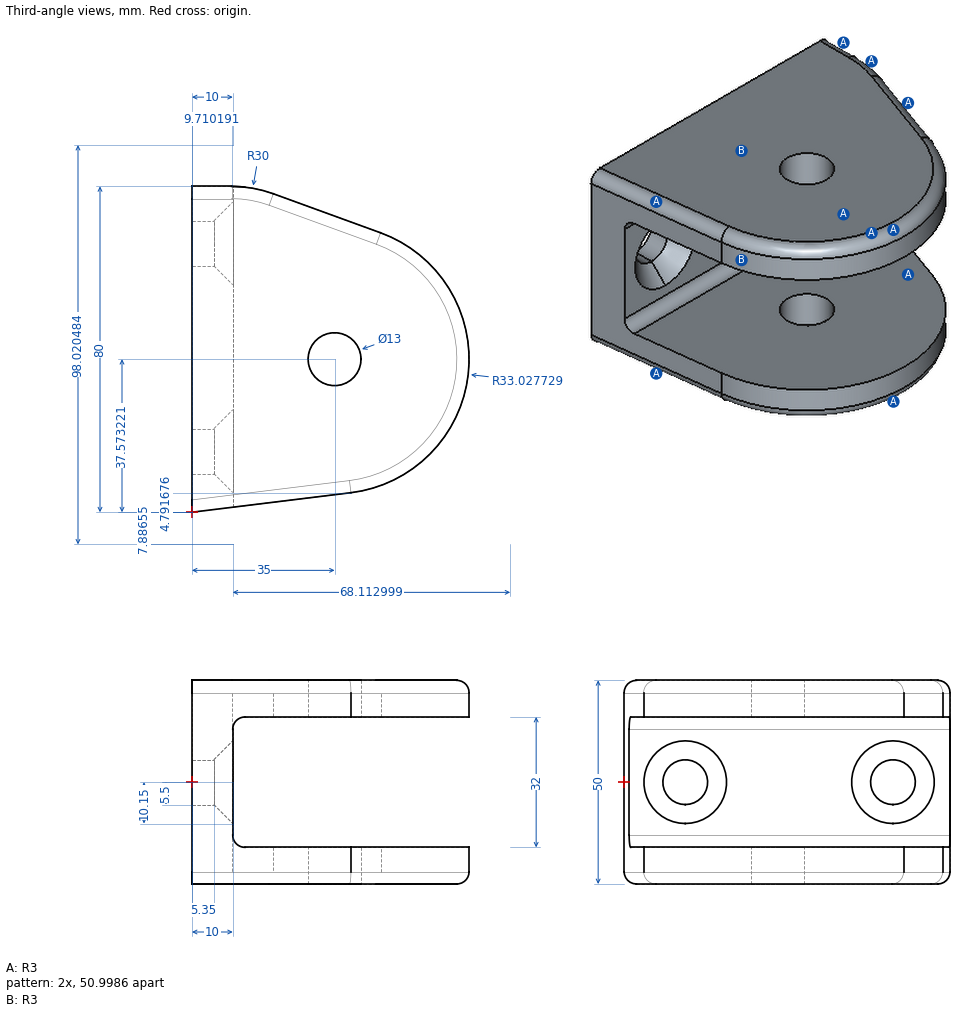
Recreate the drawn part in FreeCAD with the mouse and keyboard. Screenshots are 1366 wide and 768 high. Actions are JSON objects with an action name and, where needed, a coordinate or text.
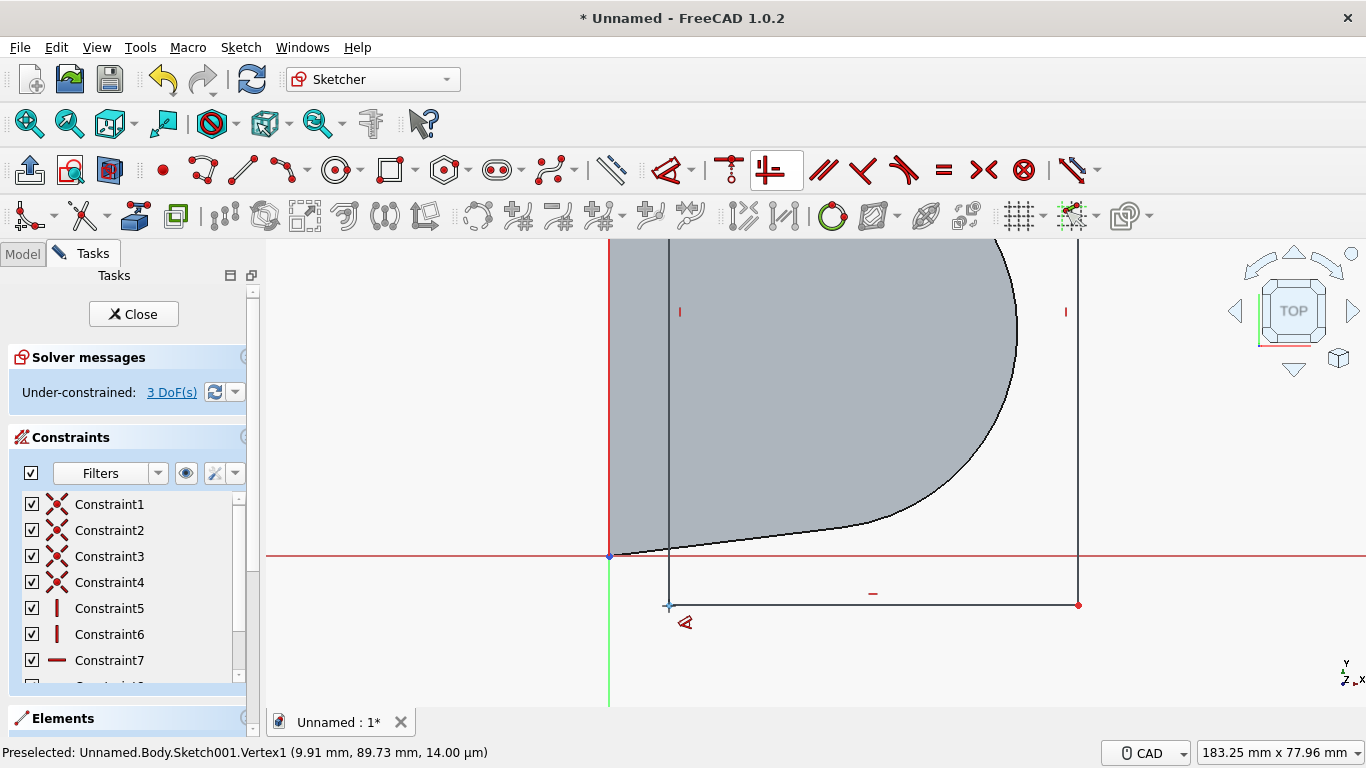
{"action": "left_click", "coordinate": [669, 605]}
{"action": "left_click", "coordinate": [575, 581]}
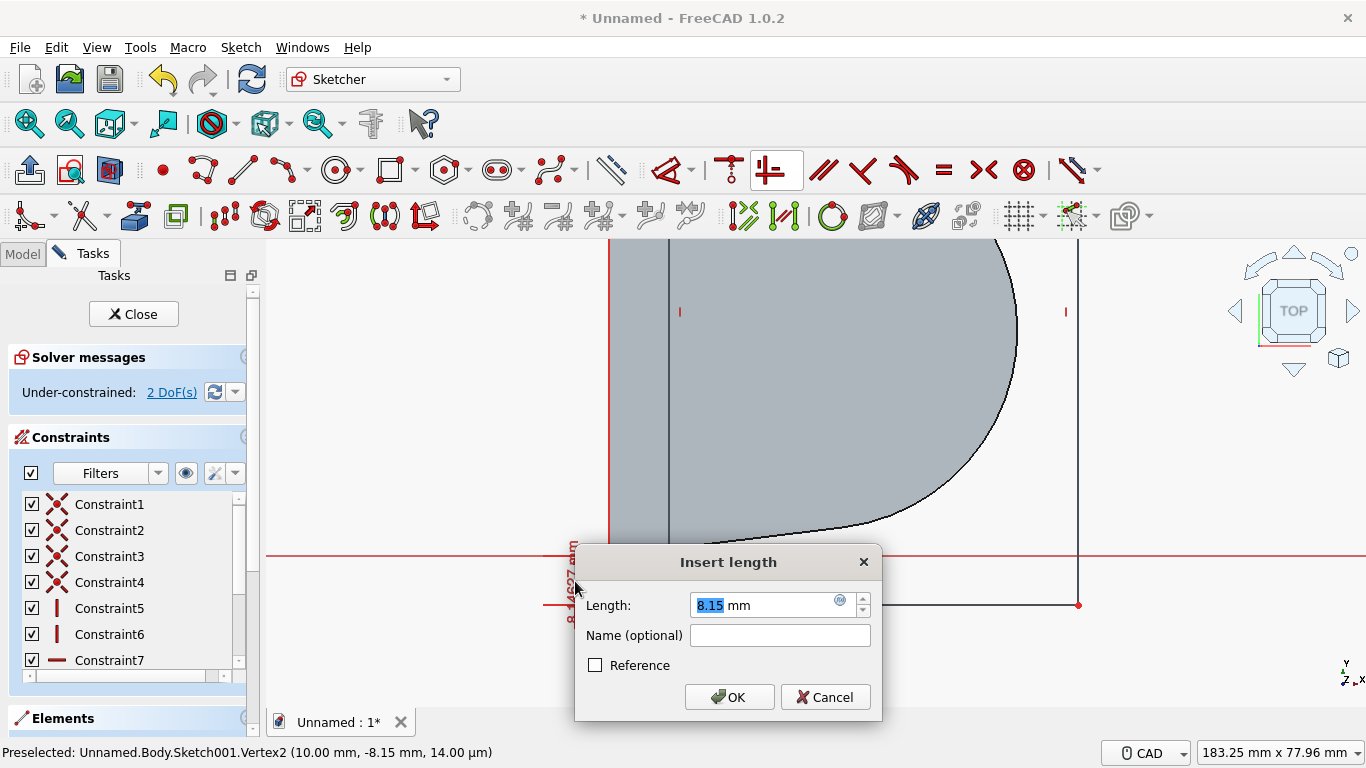
{"action": "type", "text": "7.88655"}
{"action": "key", "text": "Return"}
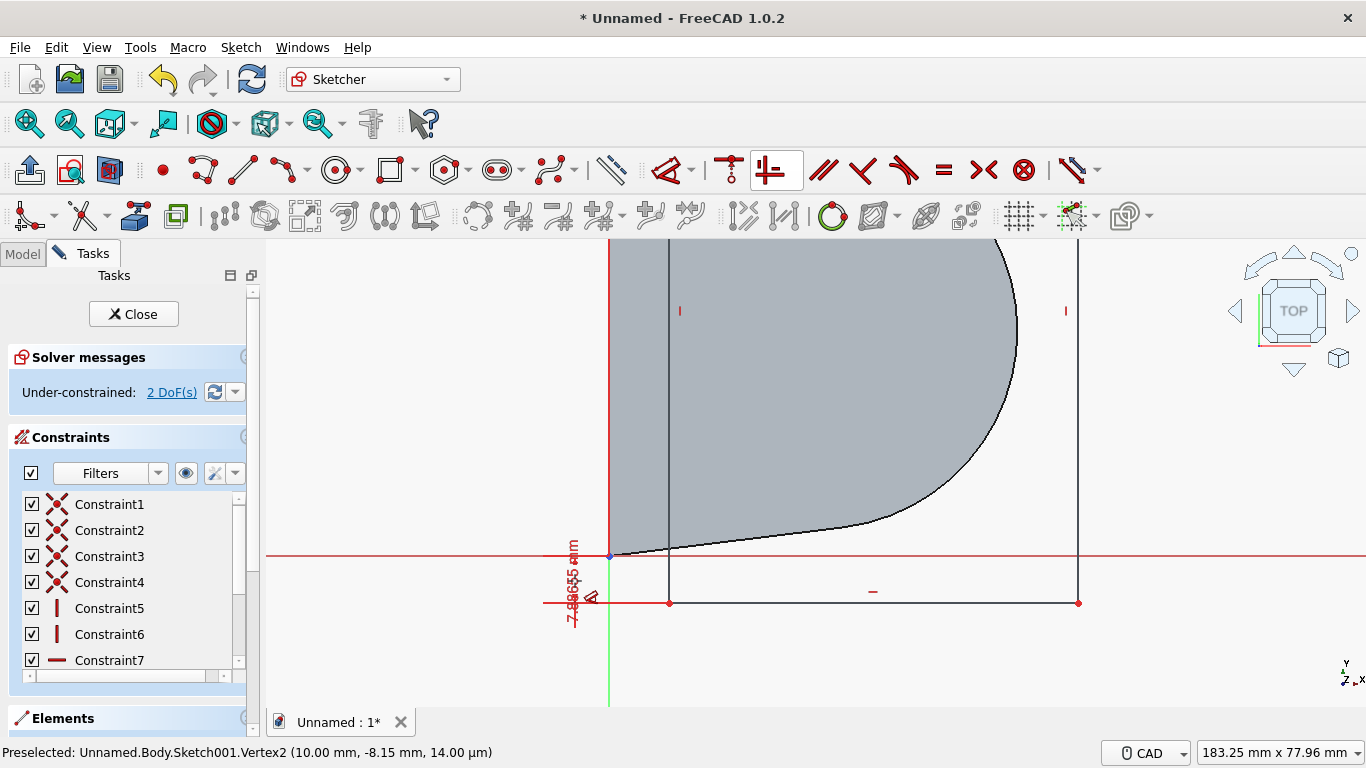
{"action": "left_click", "coordinate": [669, 428]}
{"action": "left_click", "coordinate": [635, 435]}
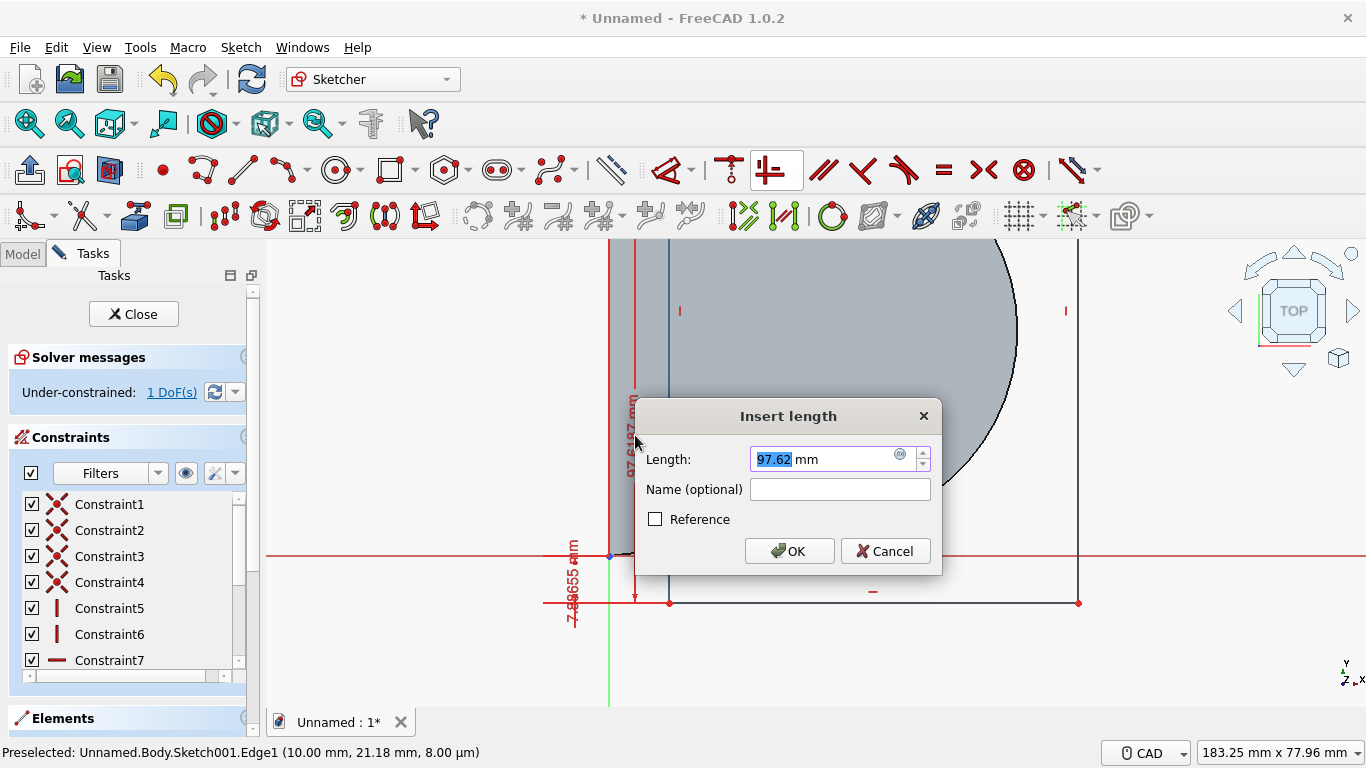
{"action": "type", "text": "98.020484"}
{"action": "key", "text": "Return"}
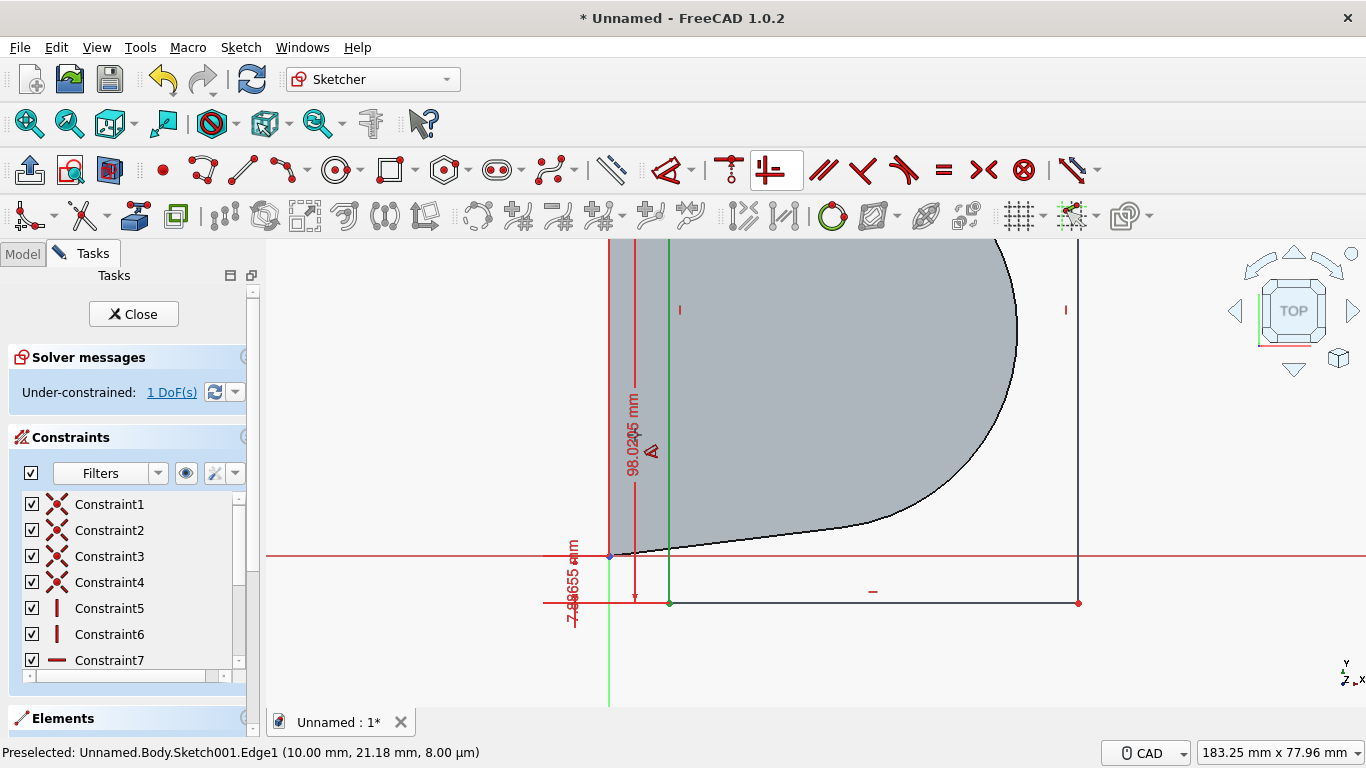
{"action": "left_click", "coordinate": [792, 603]}
{"action": "left_click", "coordinate": [874, 637]}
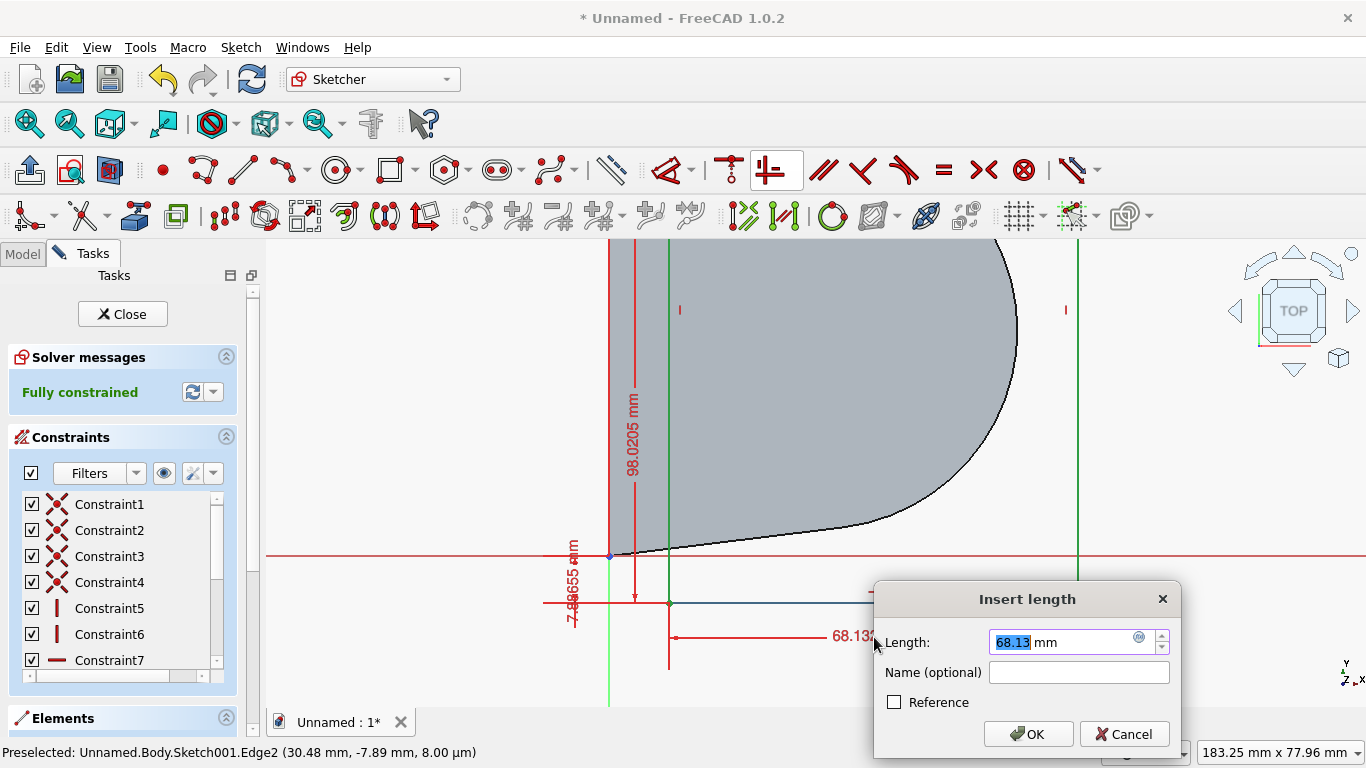
{"action": "type", "text": "68.112999"}
{"action": "key", "text": "Return"}
{"action": "key", "text": "Escape"}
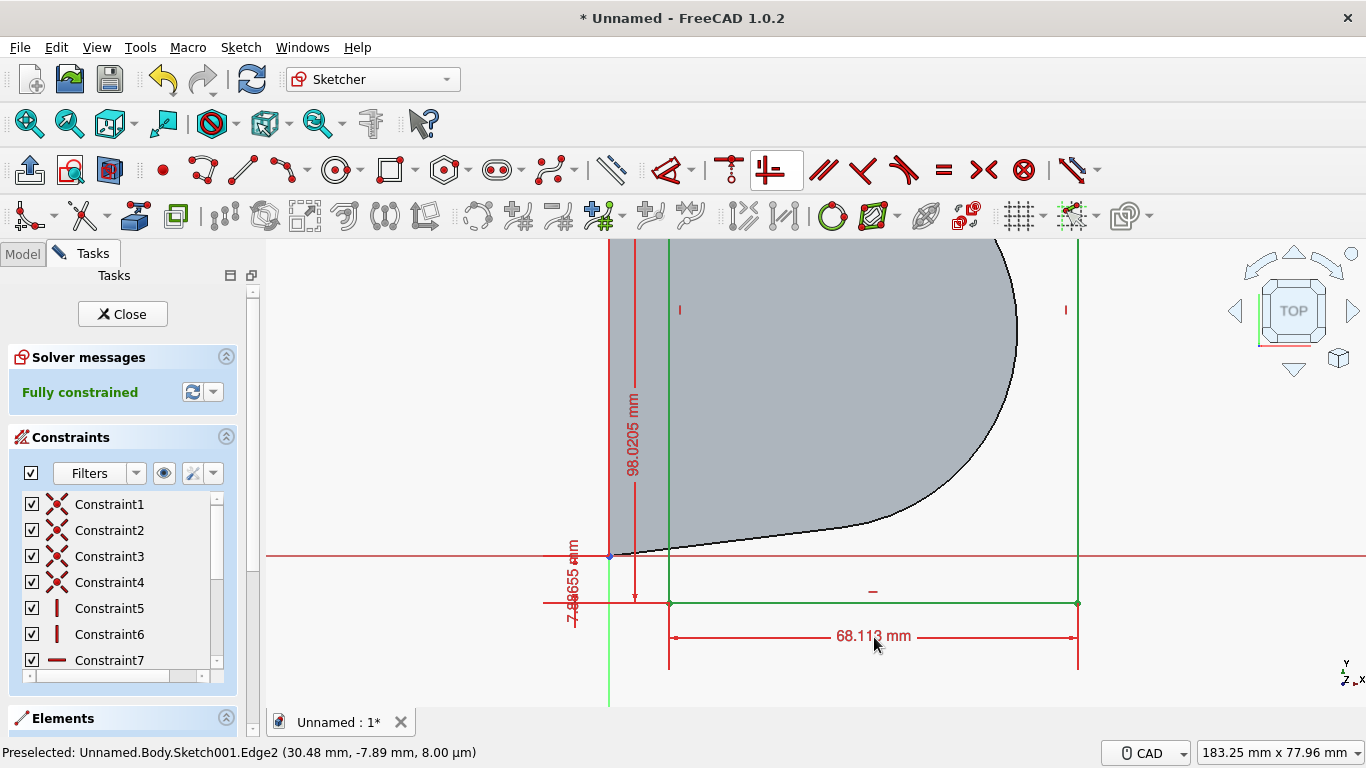
{"action": "left_click", "coordinate": [123, 314]}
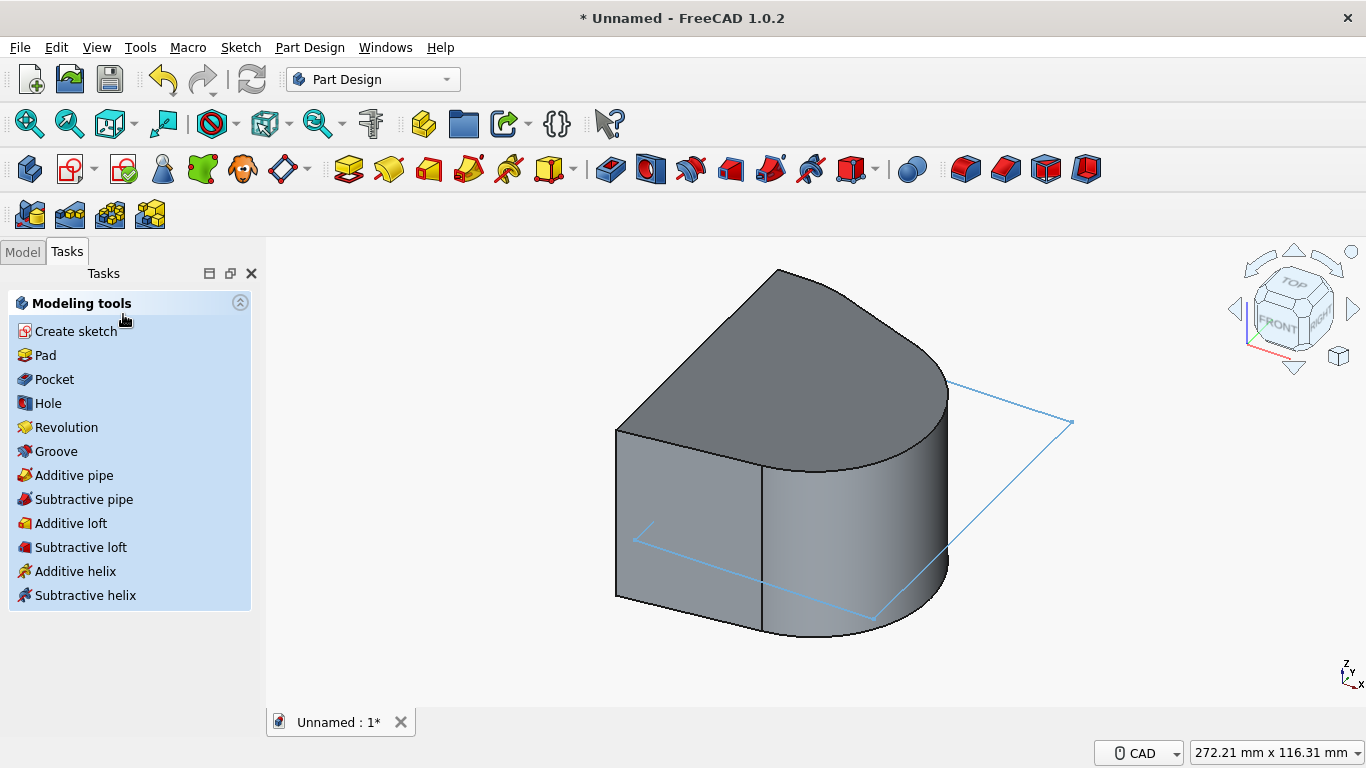
{"action": "left_click", "coordinate": [612, 170]}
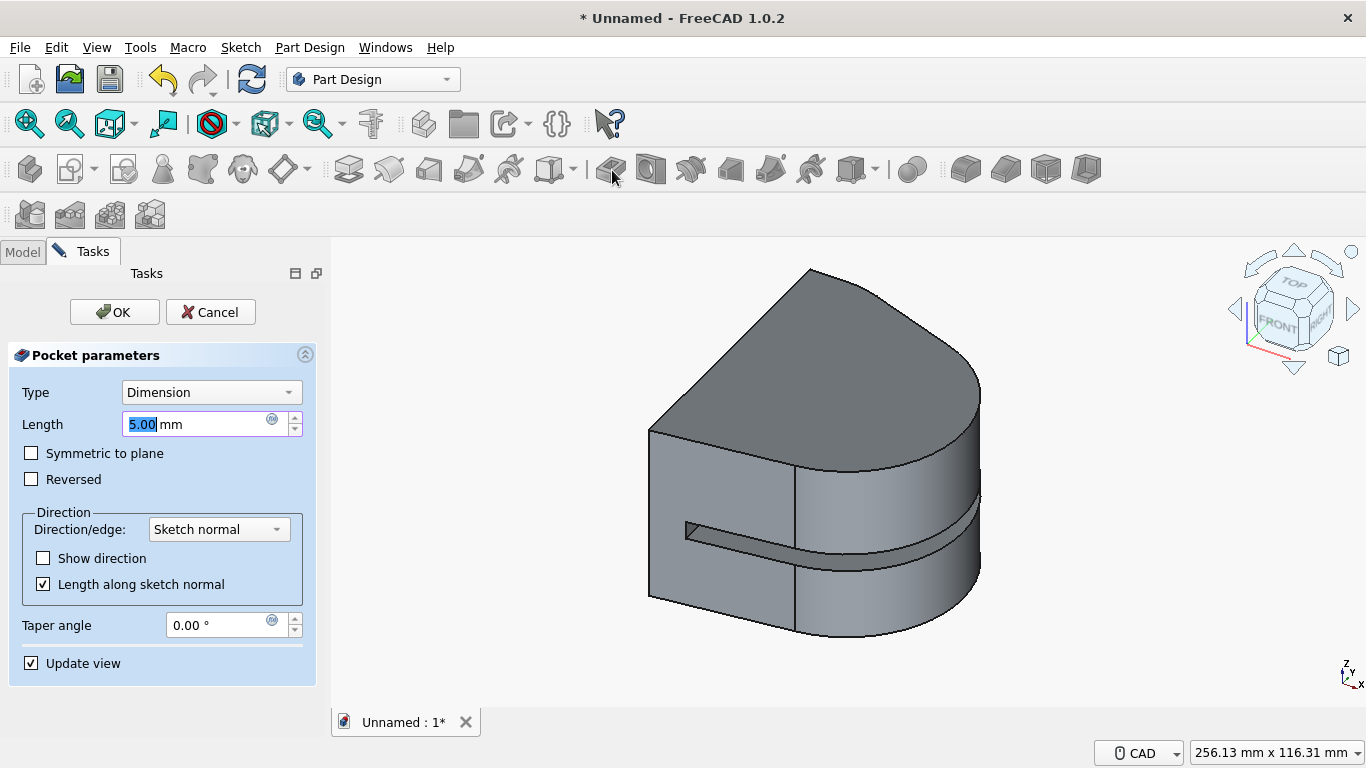
{"action": "type", "text": "32"}
{"action": "key", "text": "Tab"}